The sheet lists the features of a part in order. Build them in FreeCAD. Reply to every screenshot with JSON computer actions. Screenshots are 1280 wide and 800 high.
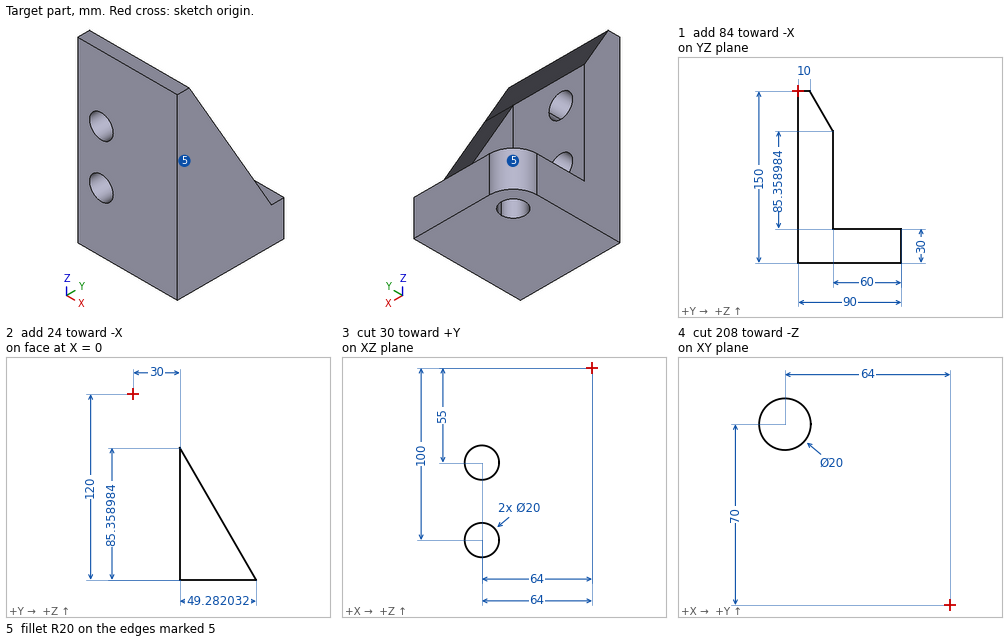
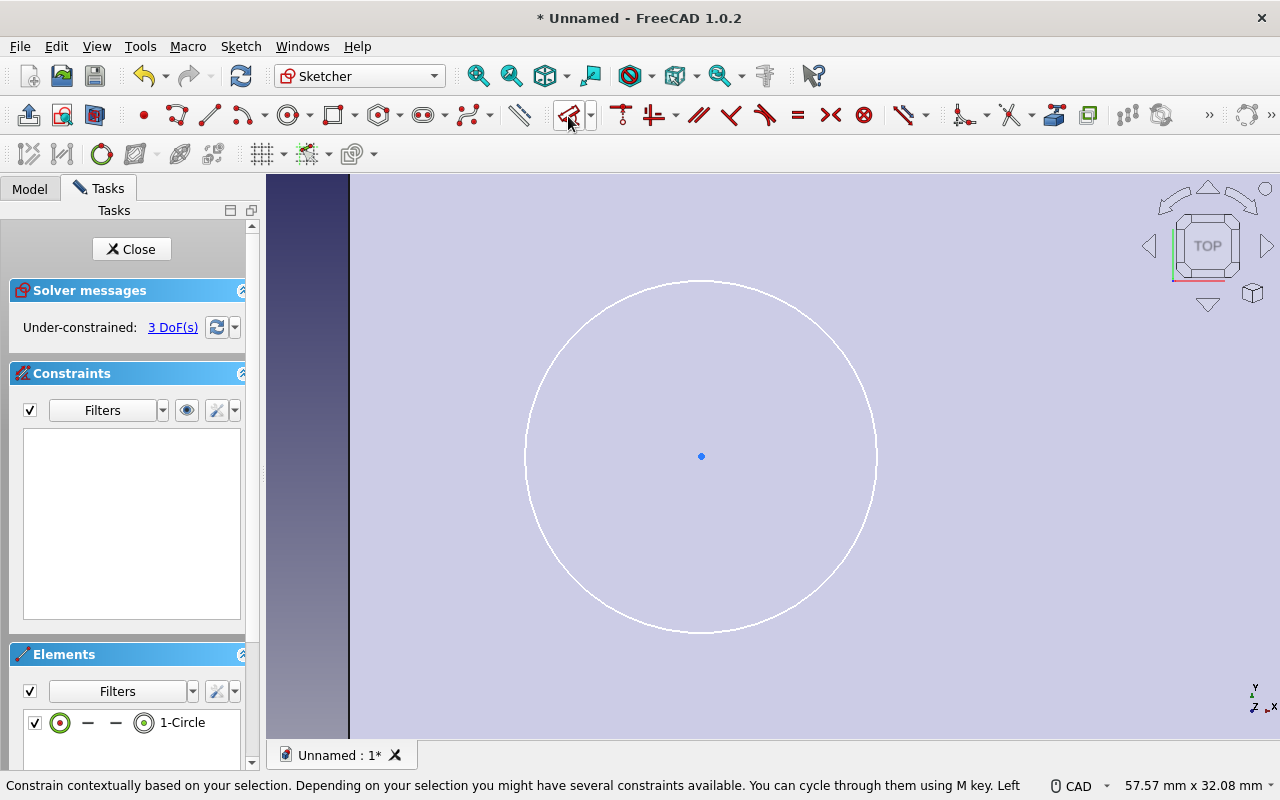
{"action": "left_click", "coordinate": [825, 332]}
{"action": "left_click", "coordinate": [848, 309]}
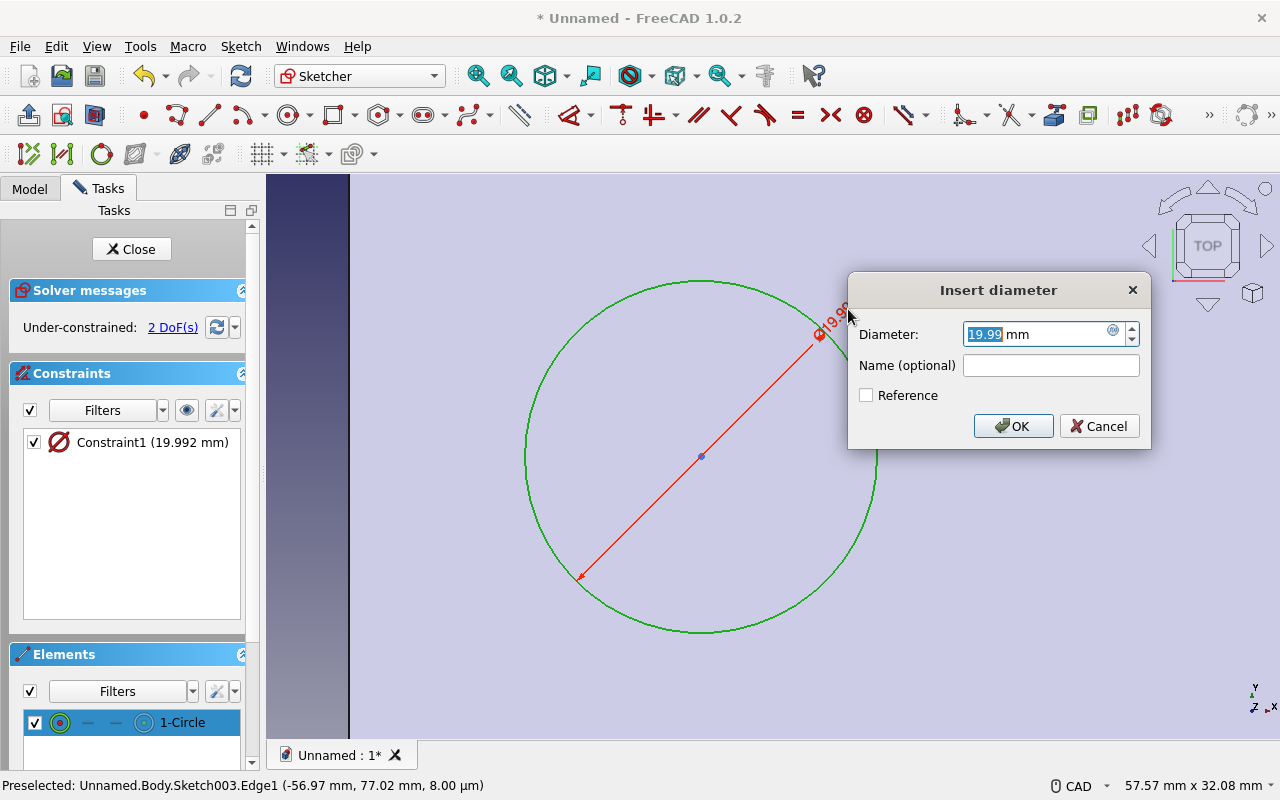
{"action": "type", "text": "20"}
{"action": "key", "text": "Return"}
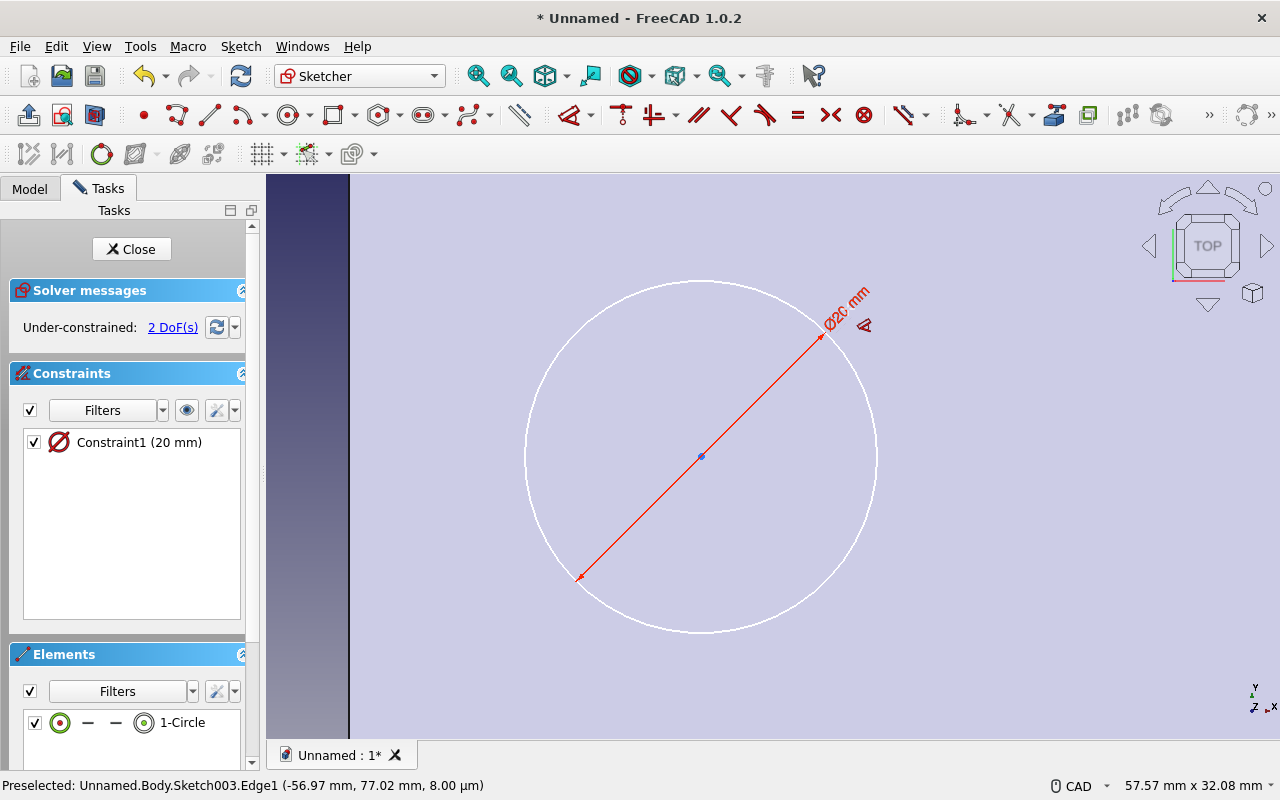
{"action": "left_click", "coordinate": [701, 457]}
{"action": "left_click", "coordinate": [908, 423]}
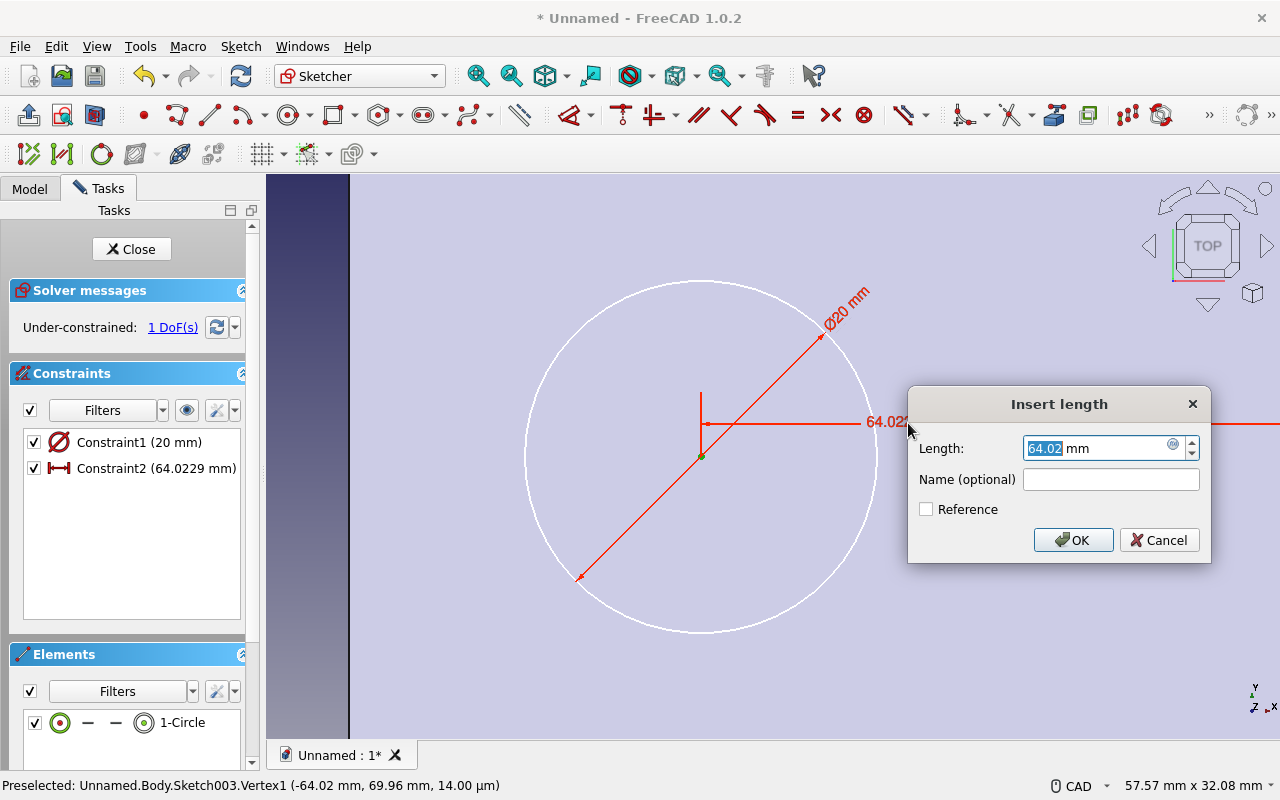
{"action": "type", "text": "64"}
{"action": "key", "text": "Return"}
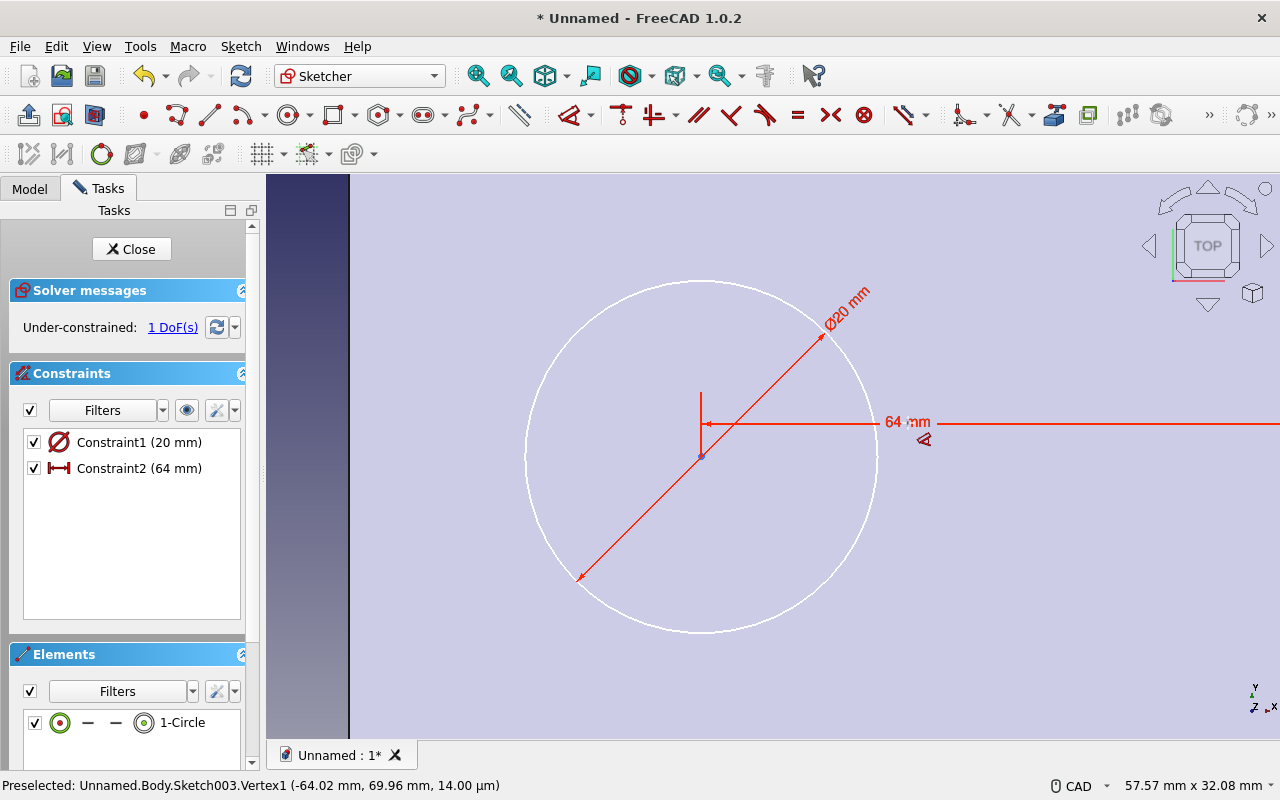
{"action": "left_click", "coordinate": [701, 457]}
{"action": "left_click", "coordinate": [667, 584]}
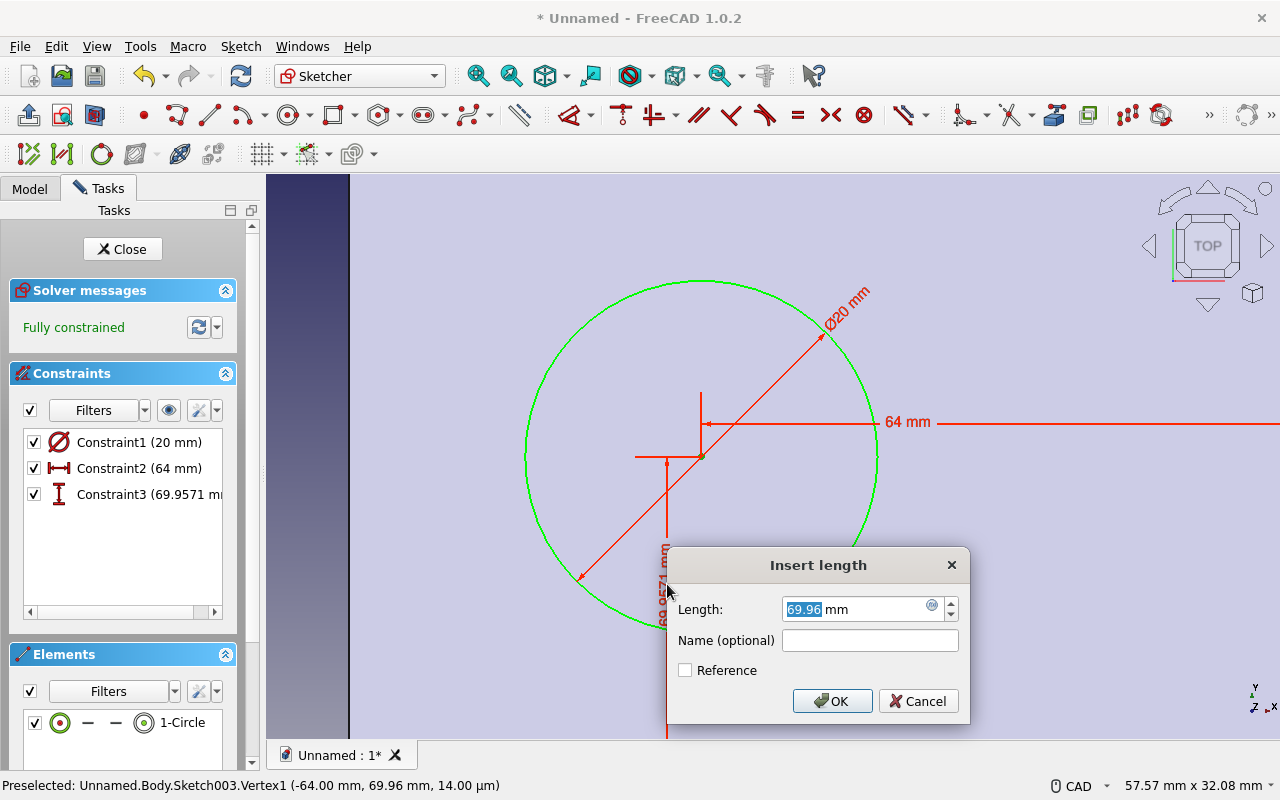
{"action": "type", "text": "70"}
{"action": "key", "text": "Return"}
{"action": "key", "text": "Escape"}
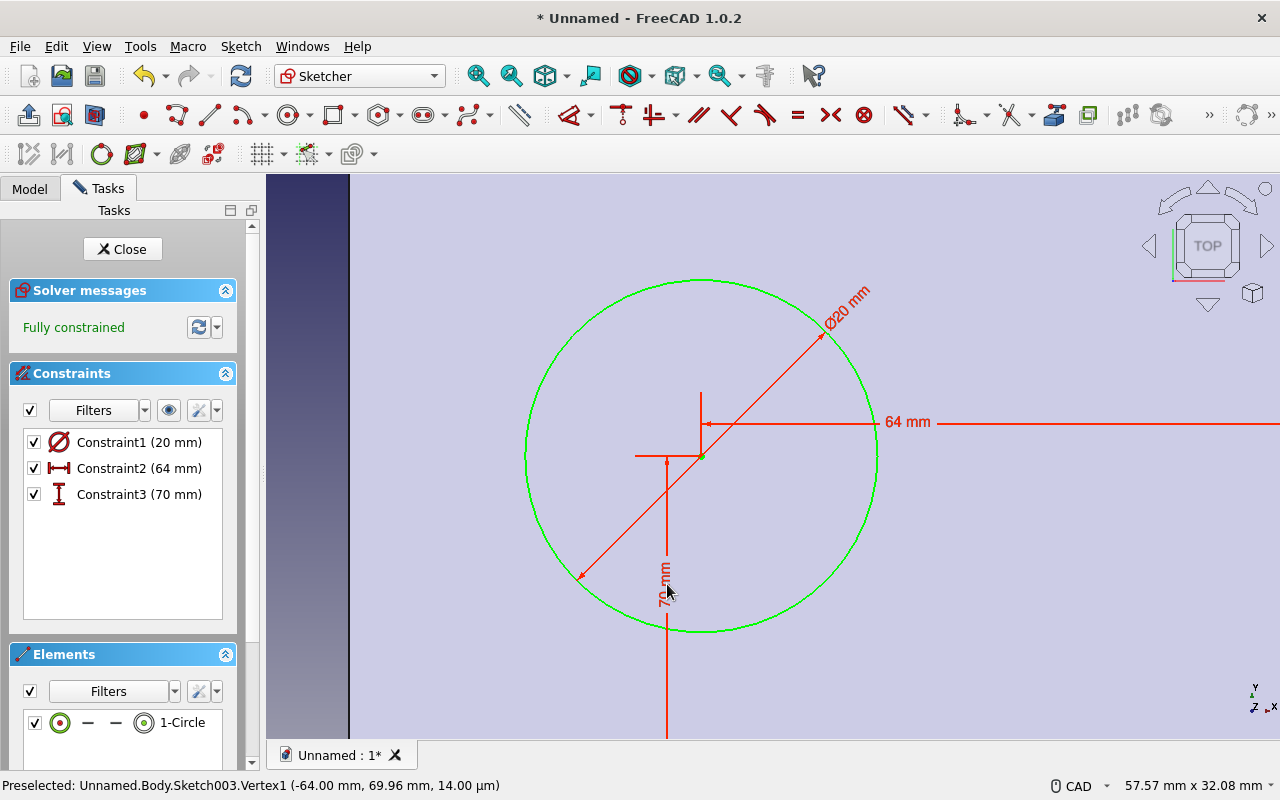
{"action": "left_click", "coordinate": [123, 249]}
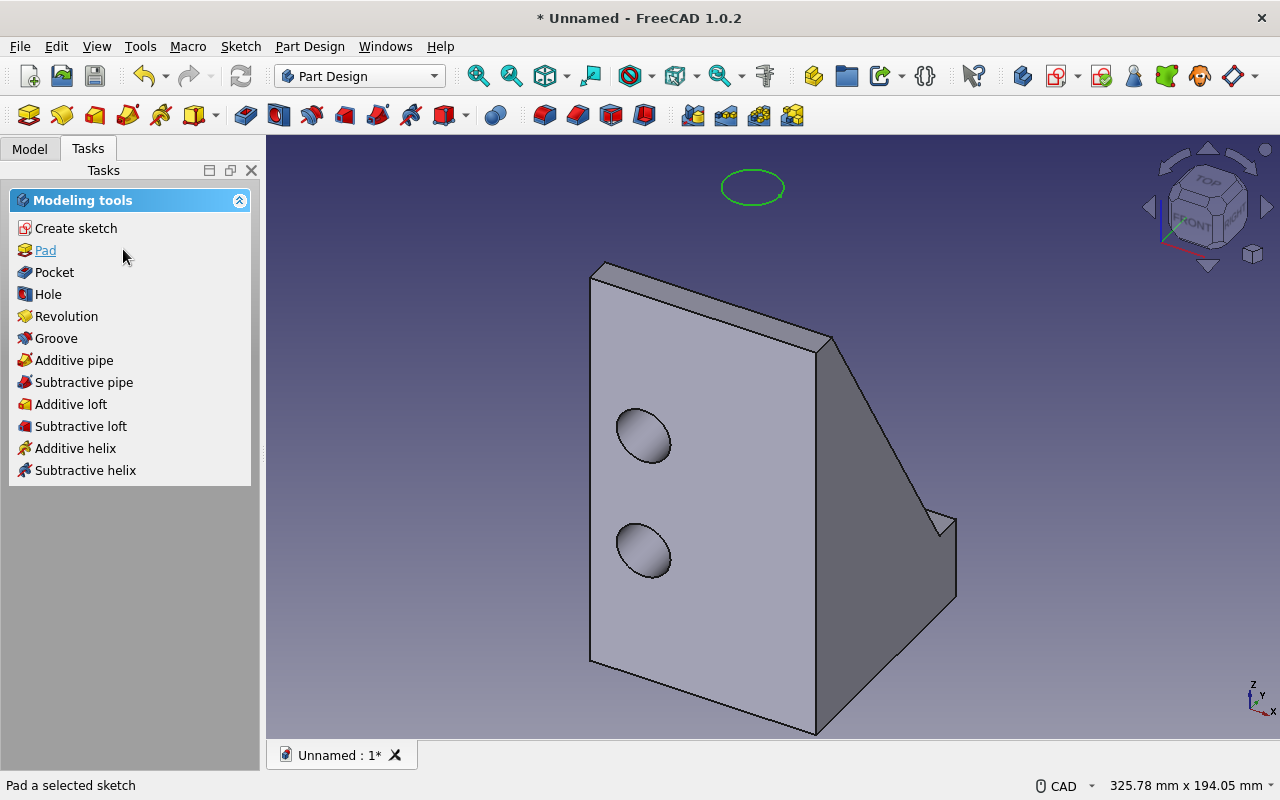
{"action": "left_click", "coordinate": [246, 116]}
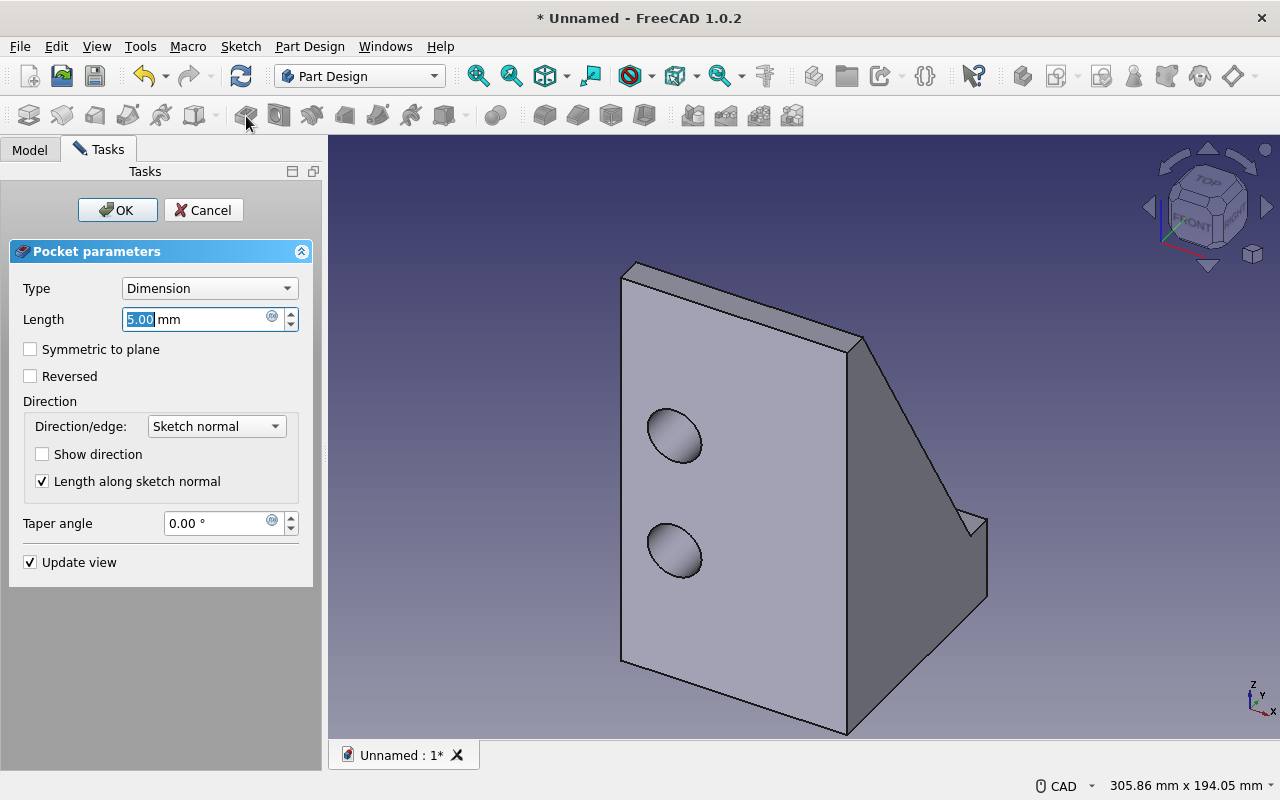
{"action": "type", "text": "208"}
{"action": "key", "text": "Tab"}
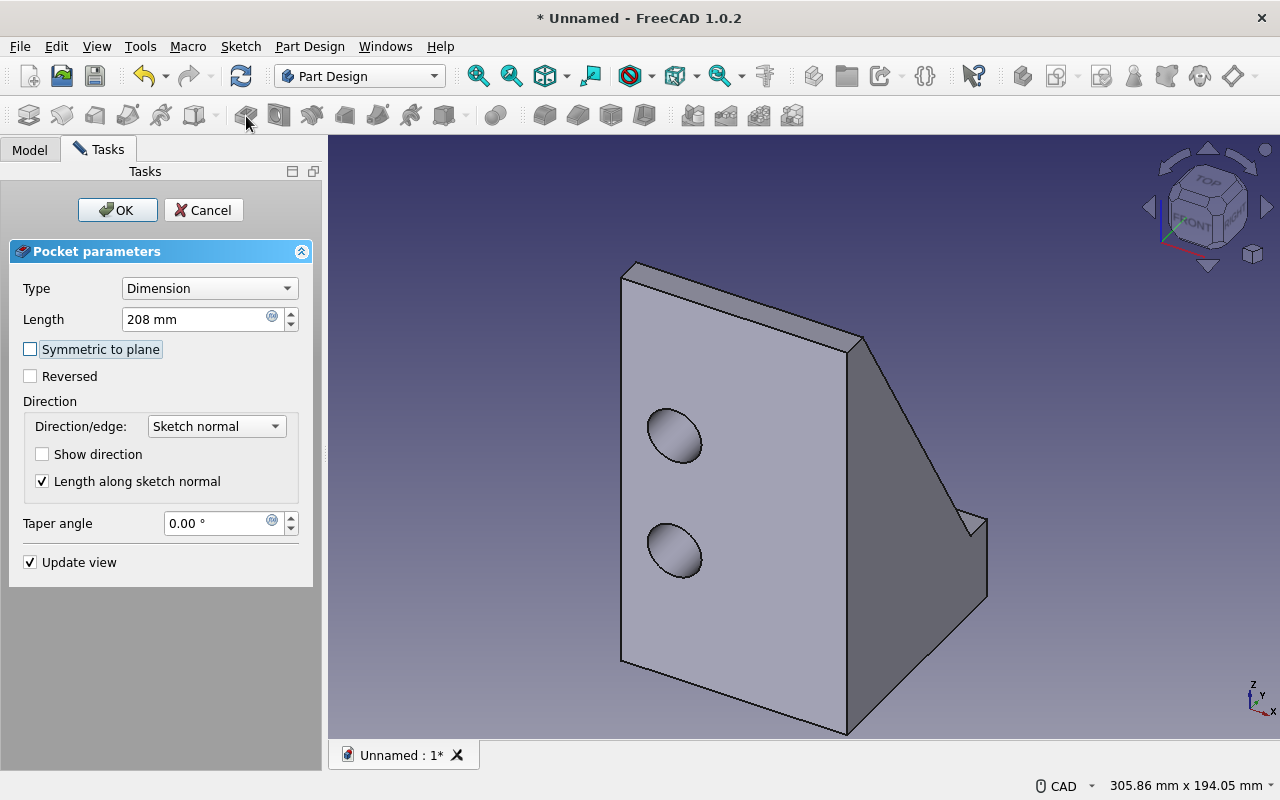
{"action": "left_click", "coordinate": [118, 210]}